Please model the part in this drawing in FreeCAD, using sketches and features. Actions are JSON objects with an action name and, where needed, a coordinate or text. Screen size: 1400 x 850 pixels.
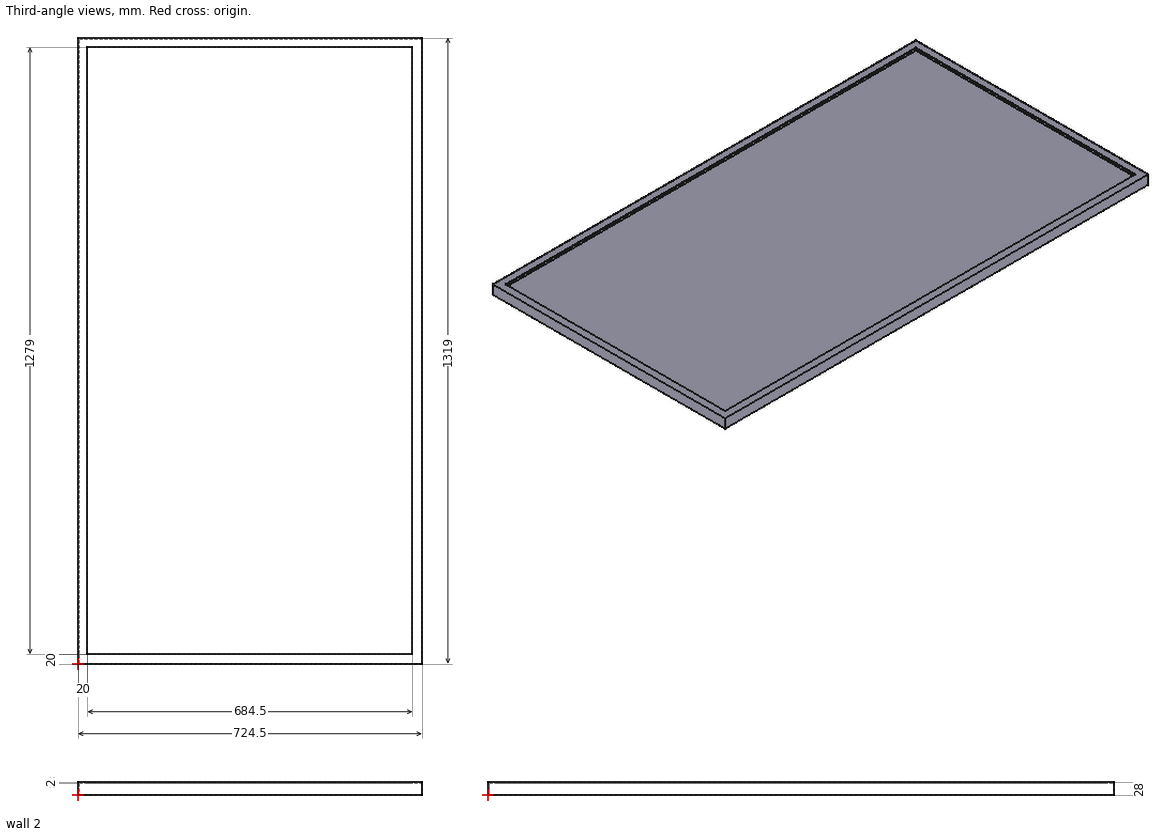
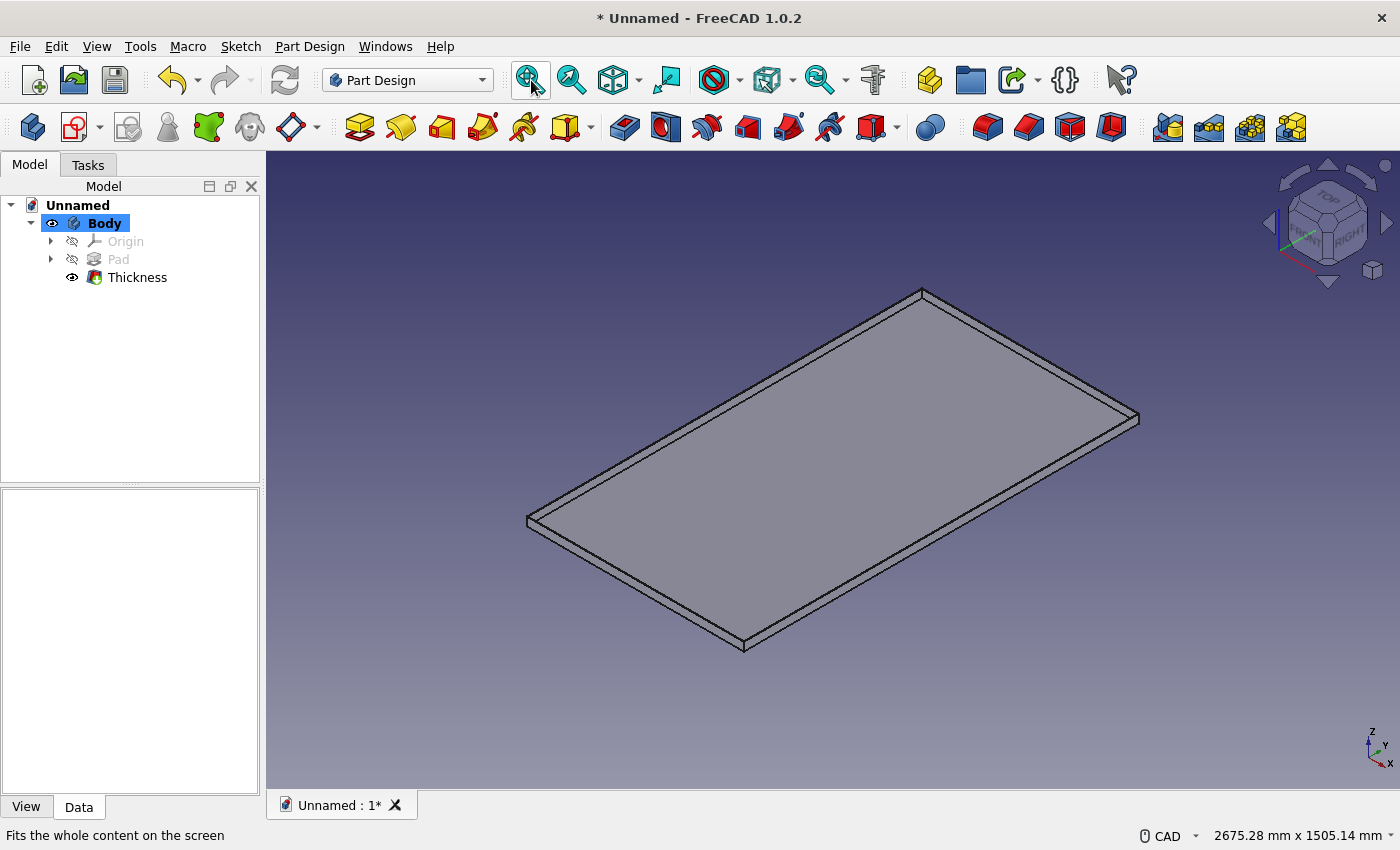
{"action": "scroll", "coordinate": [1066, 371], "scroll_direction": "up", "scroll_amount": 15}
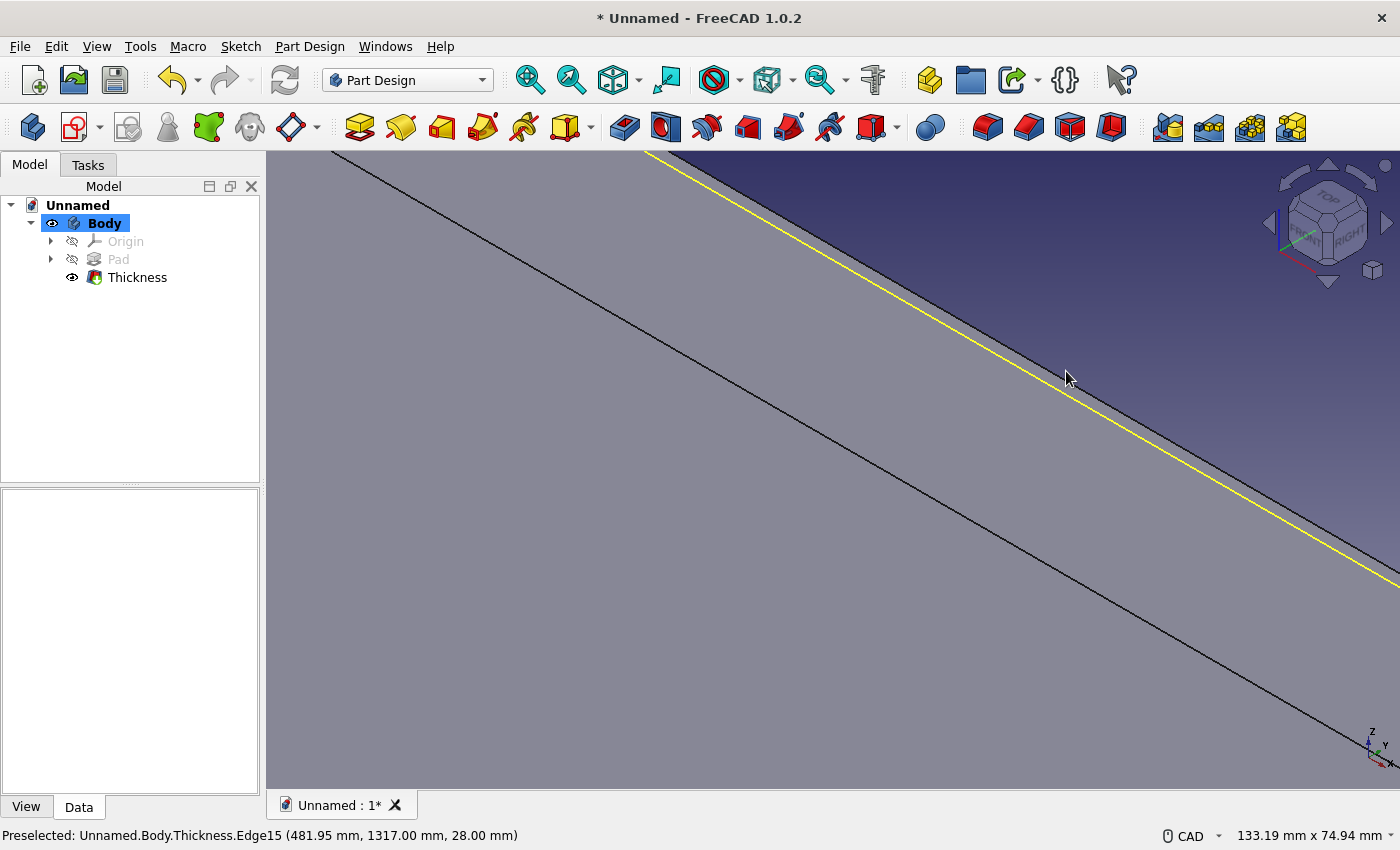
{"action": "scroll", "coordinate": [1062, 387], "scroll_direction": "up", "scroll_amount": 4}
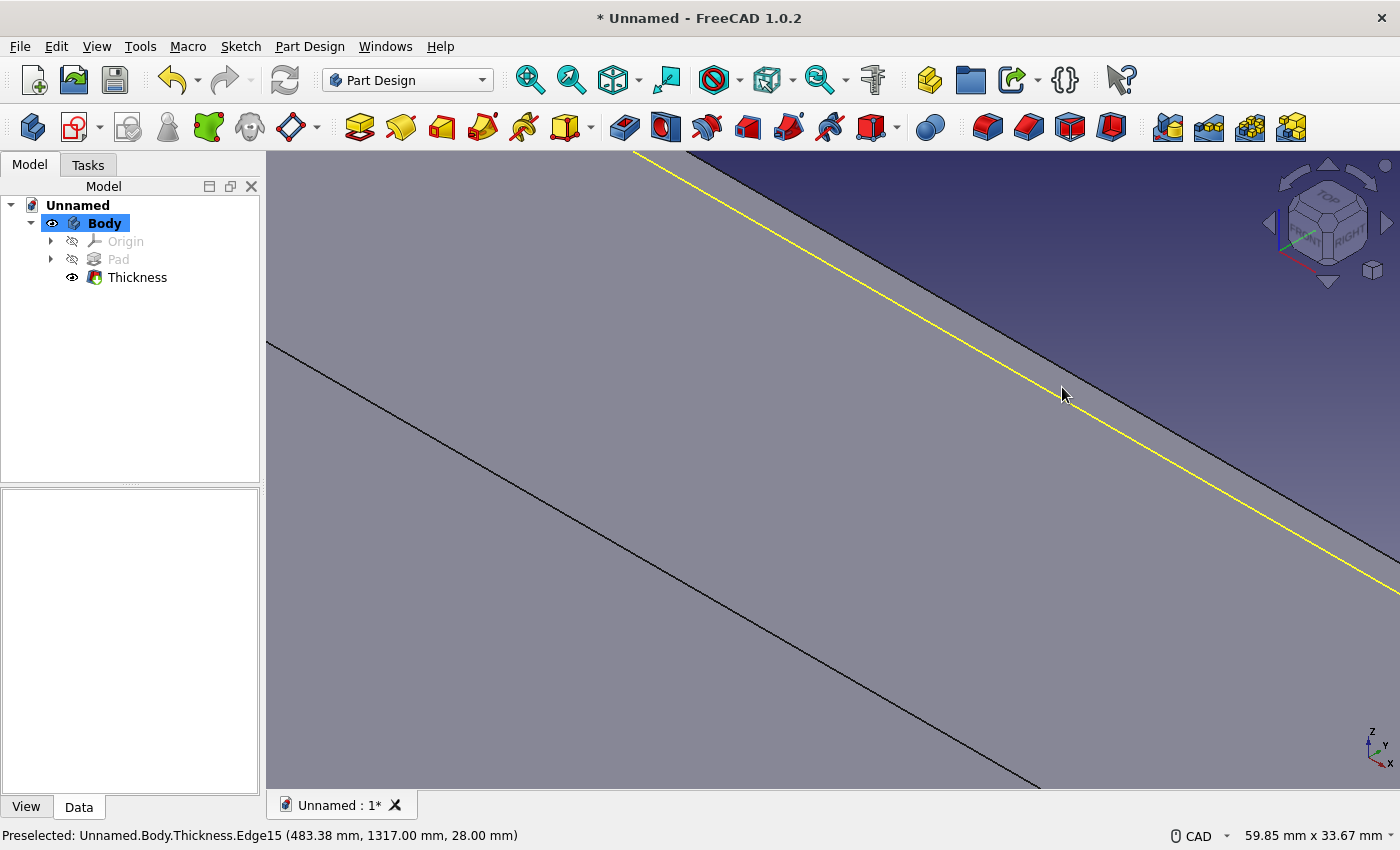
{"action": "left_click", "coordinate": [531, 80]}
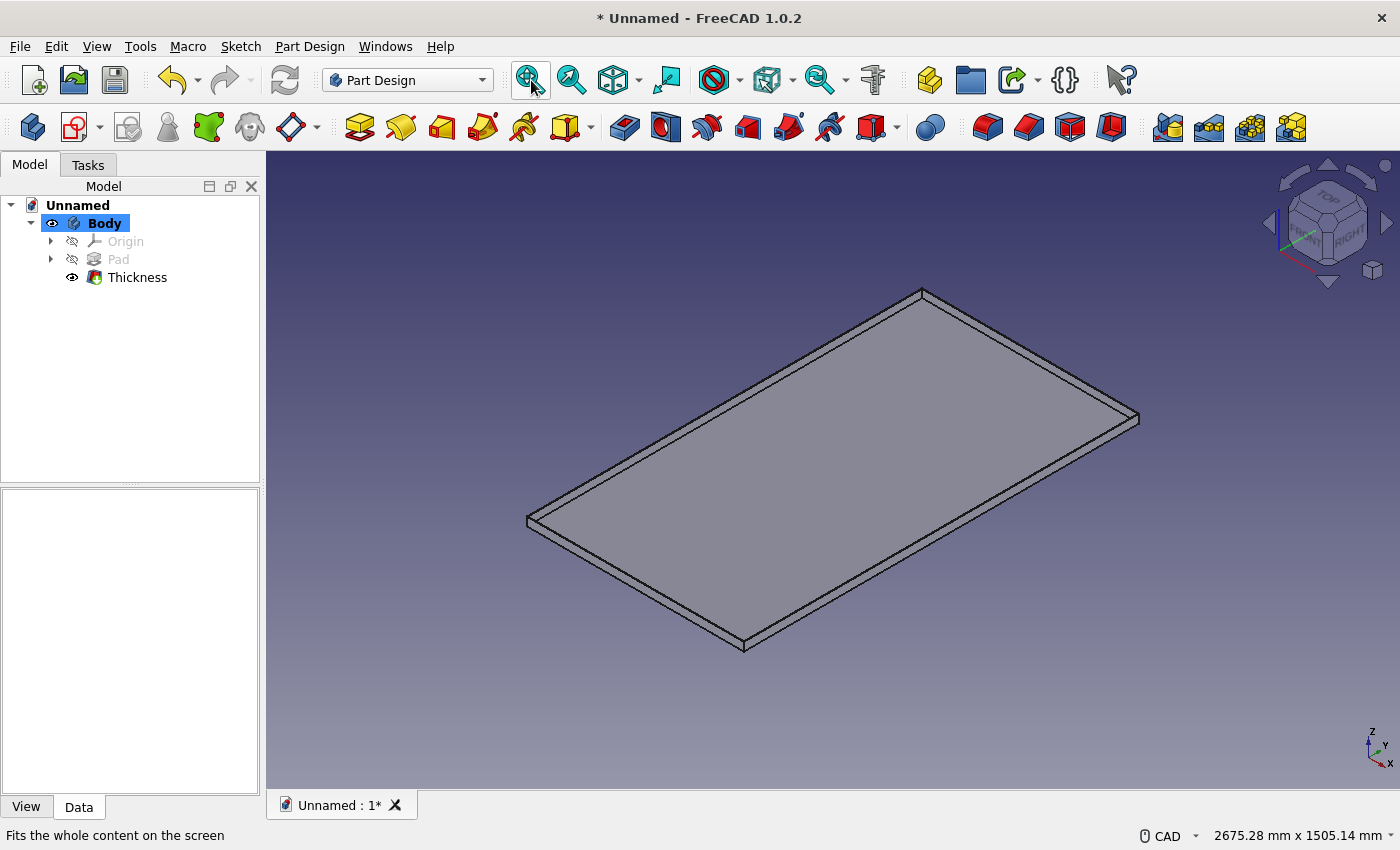
{"action": "key", "text": "2"}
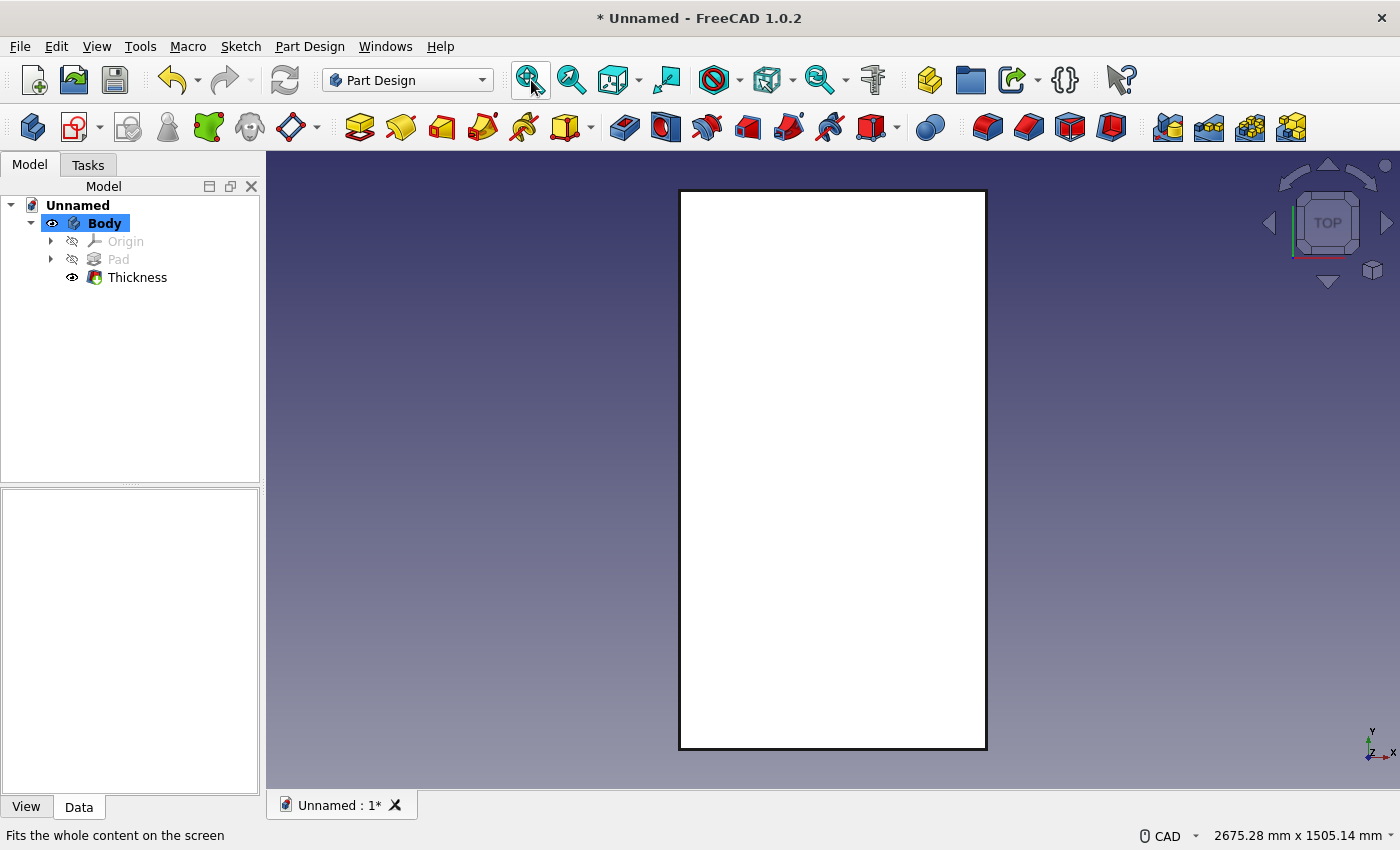
{"action": "scroll", "coordinate": [884, 190], "scroll_direction": "up", "scroll_amount": 15}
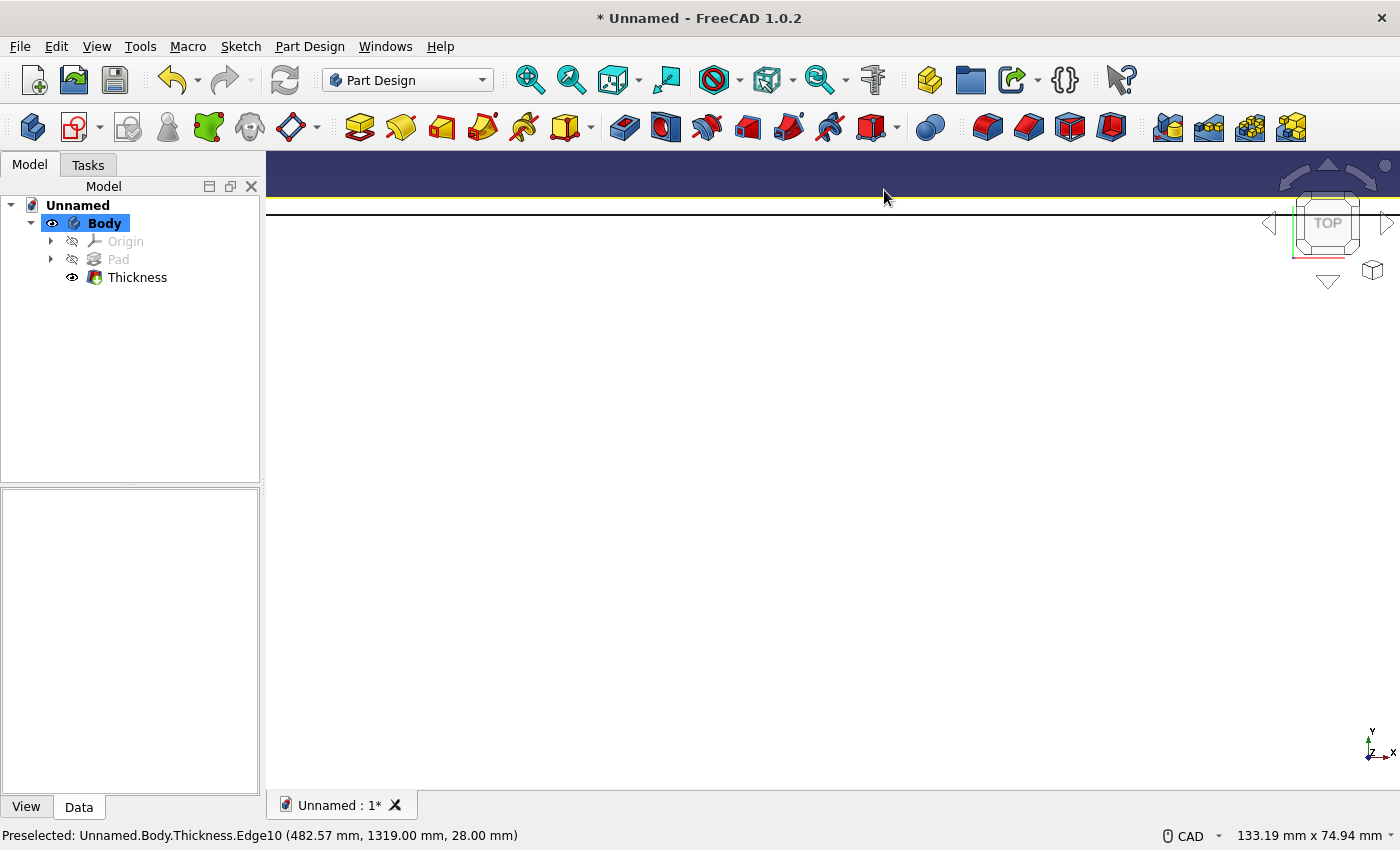
{"action": "scroll", "coordinate": [877, 208], "scroll_direction": "up", "scroll_amount": 4}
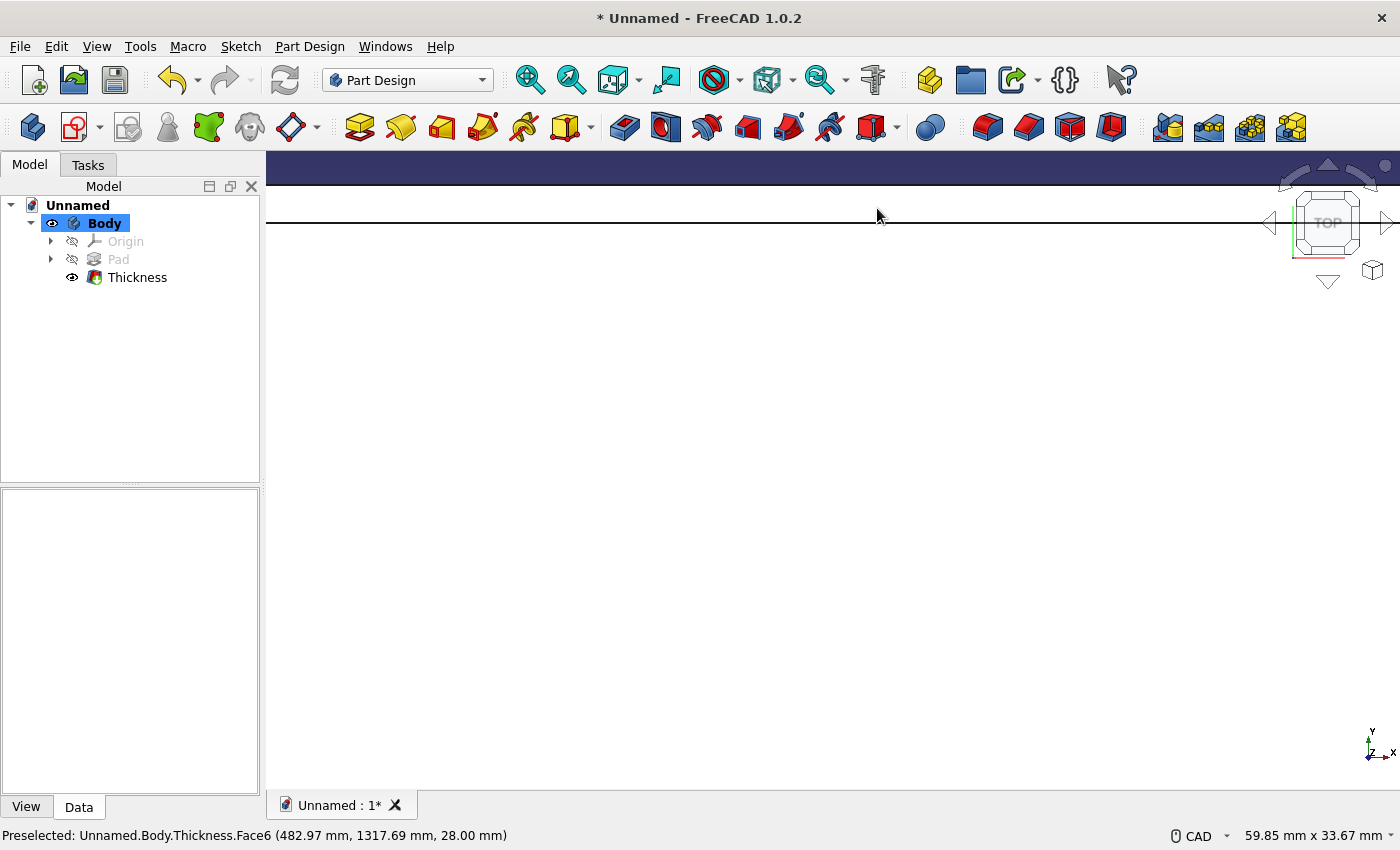
{"action": "left_click", "coordinate": [877, 210]}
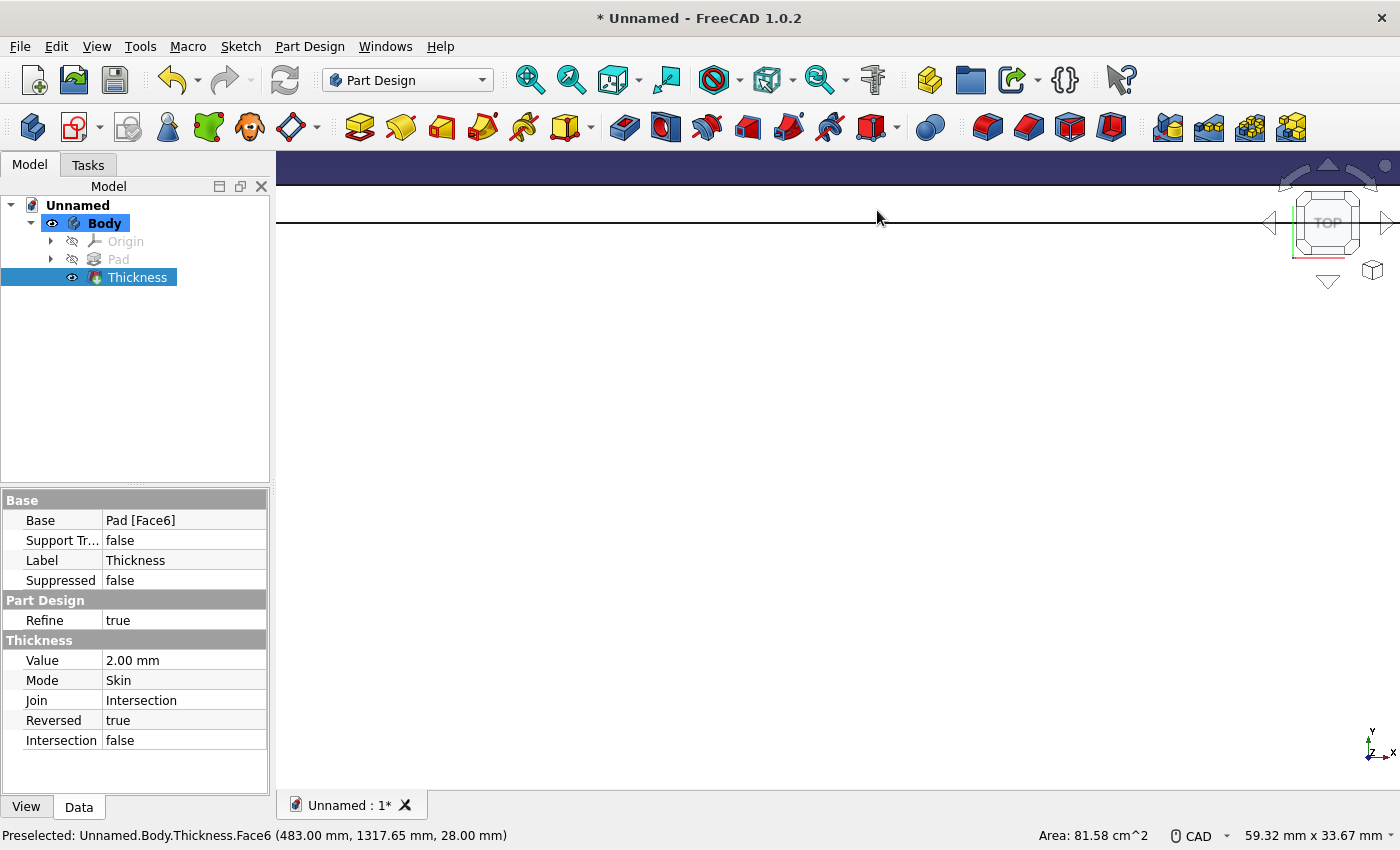
{"action": "left_click", "coordinate": [74, 128]}